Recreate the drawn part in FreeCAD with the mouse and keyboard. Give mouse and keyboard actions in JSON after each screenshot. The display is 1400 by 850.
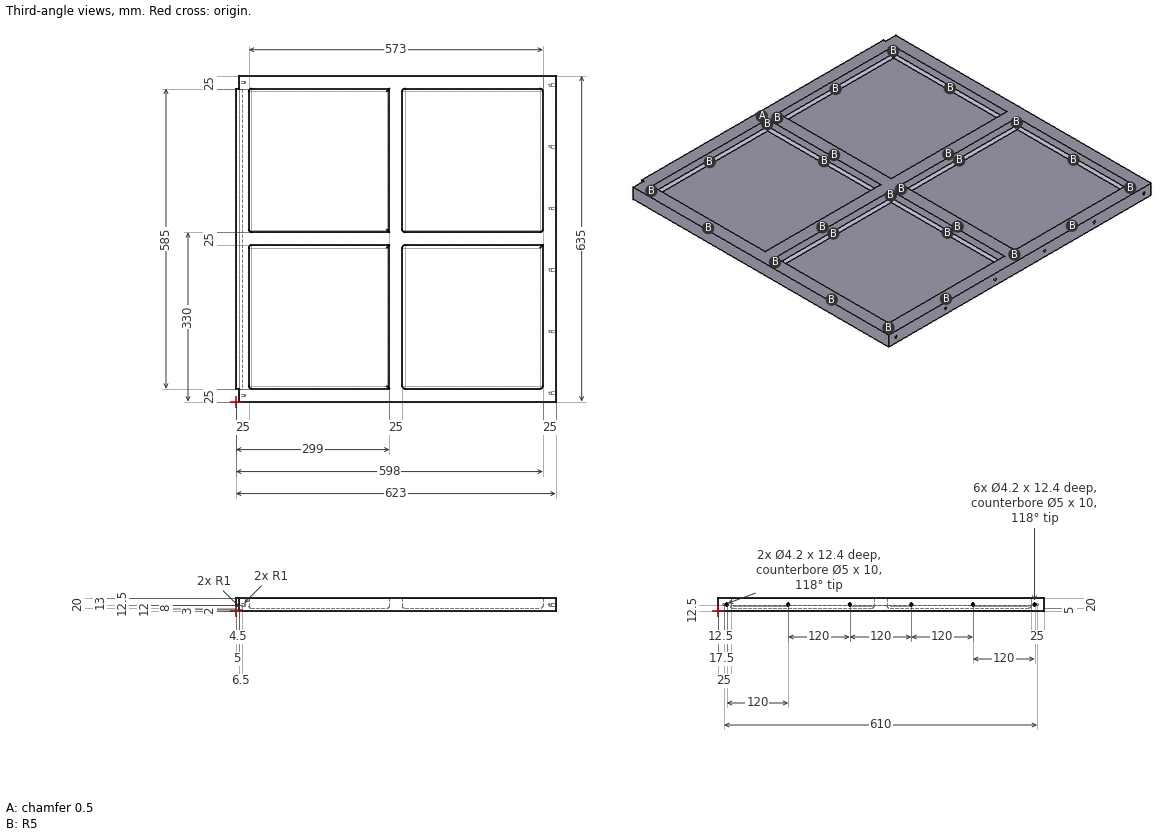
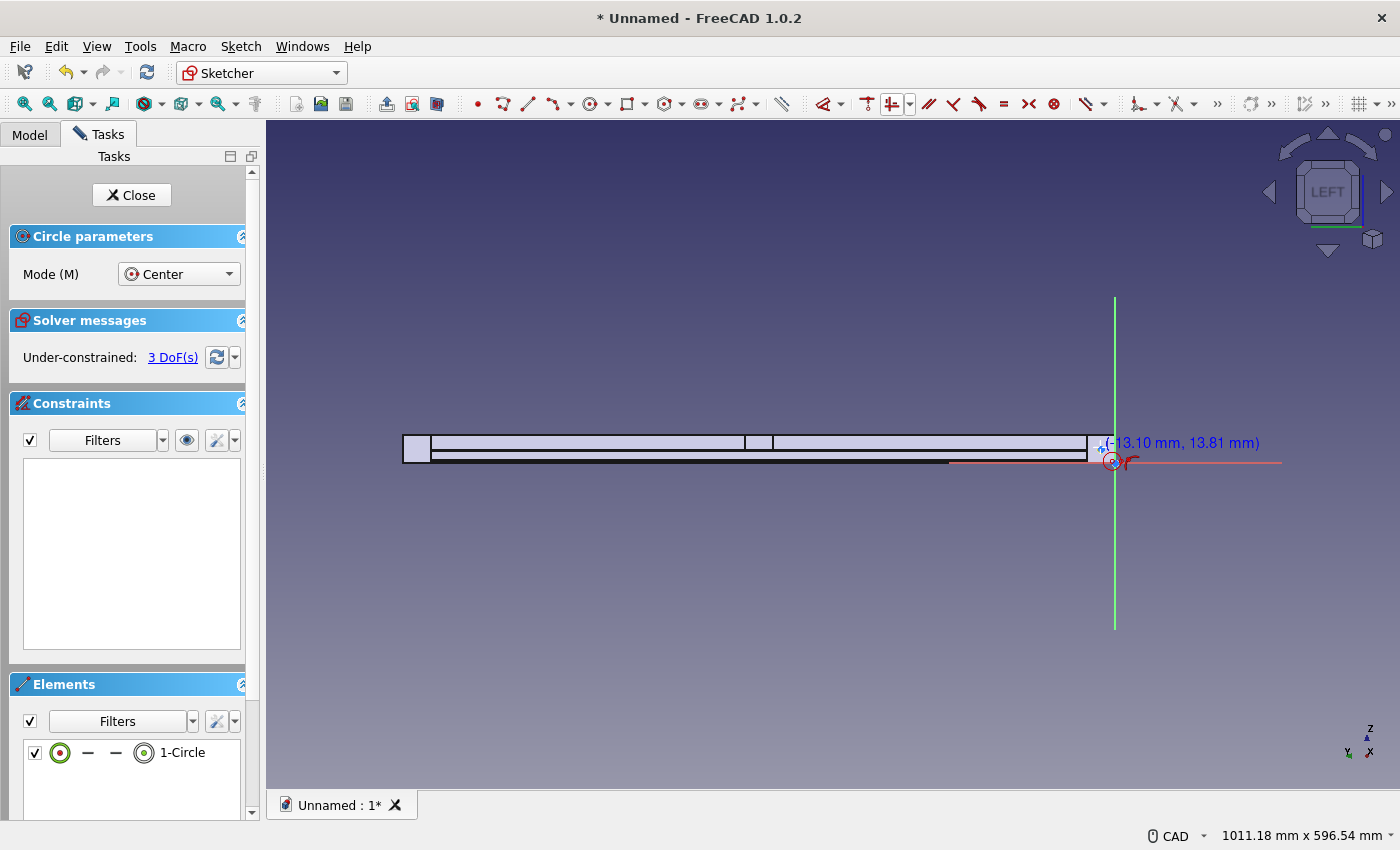
{"action": "scroll", "coordinate": [417, 449], "scroll_direction": "up", "scroll_amount": 12}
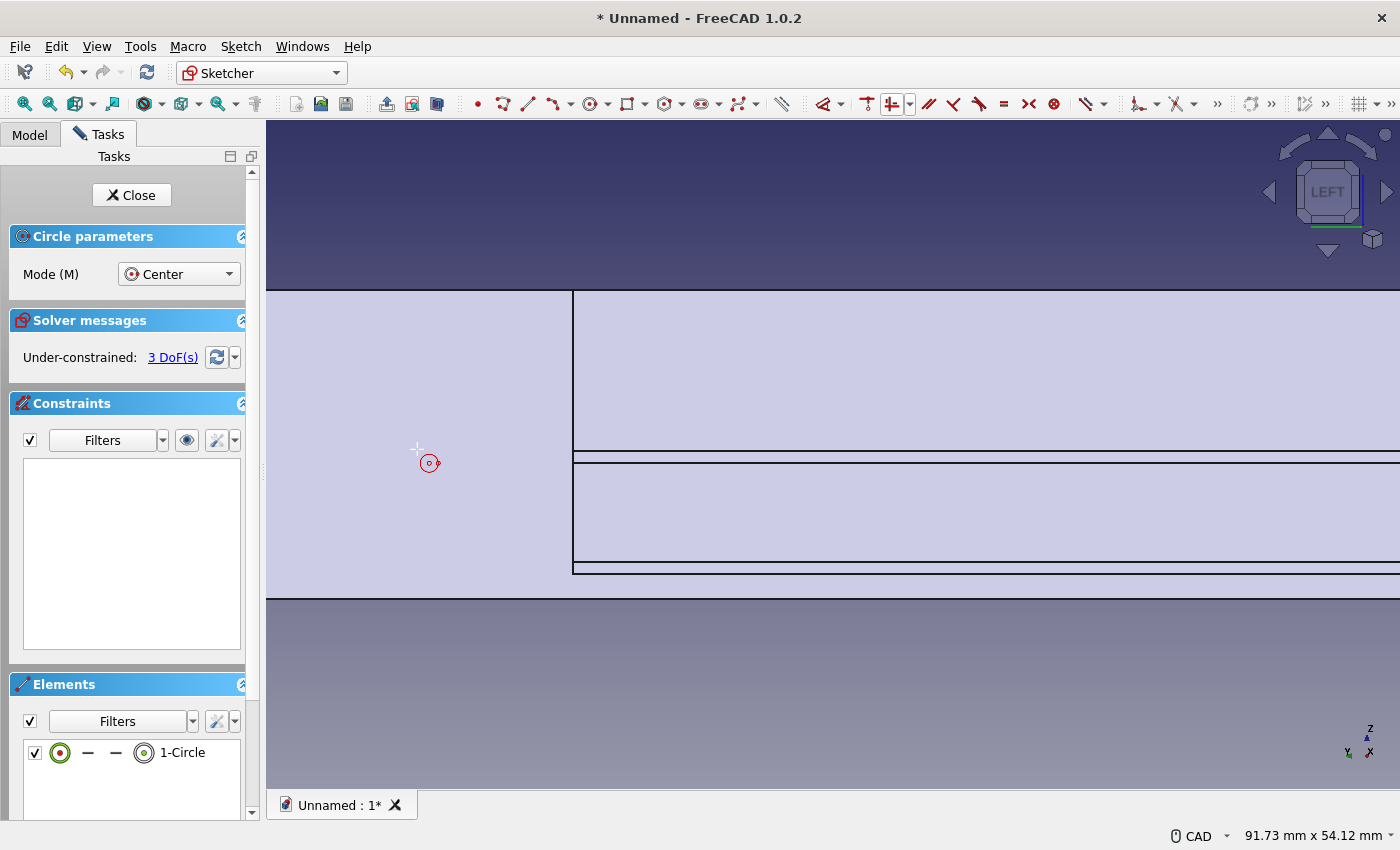
{"action": "scroll", "coordinate": [416, 449], "scroll_direction": "down", "scroll_amount": 12}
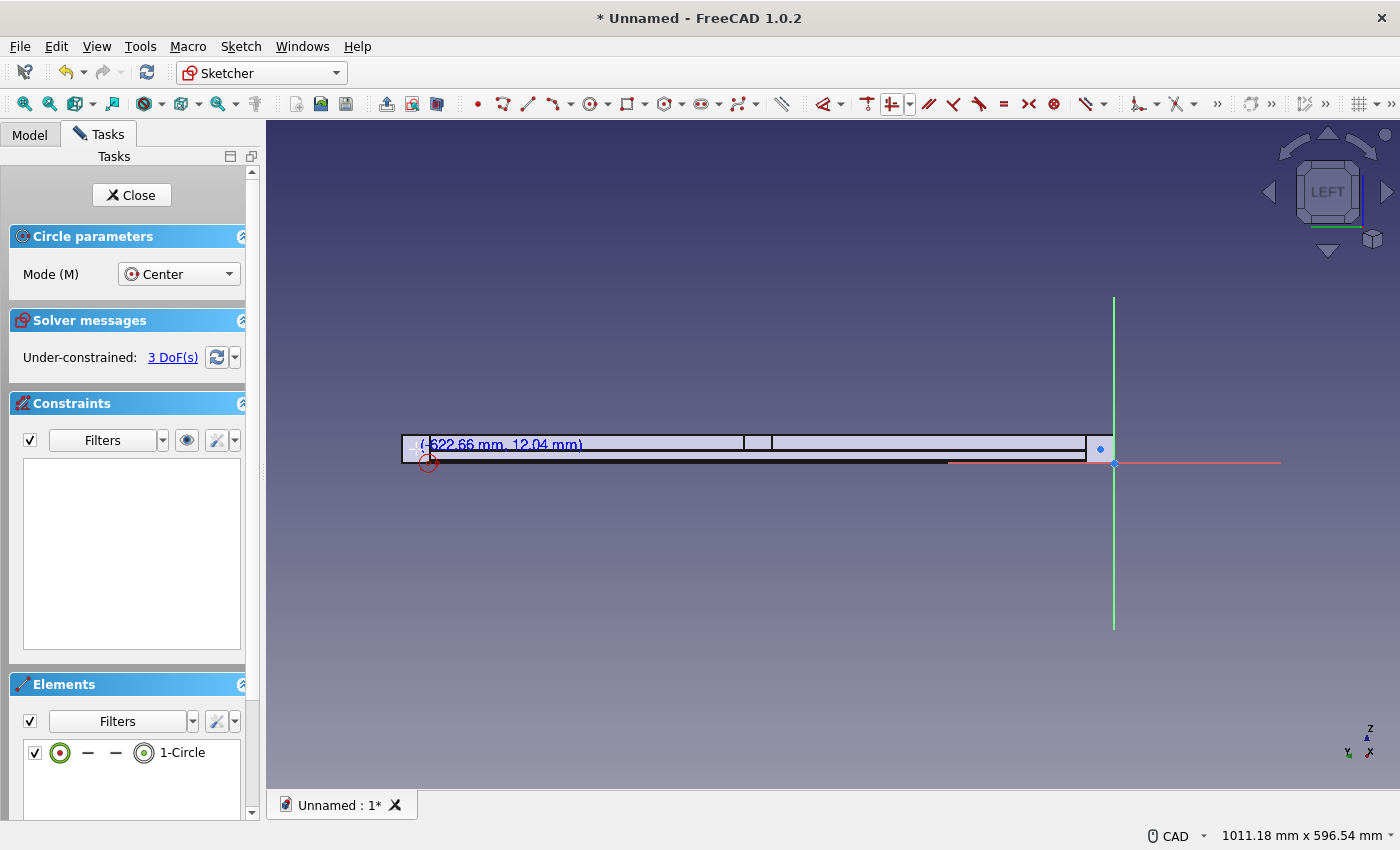
{"action": "left_click", "coordinate": [416, 449]}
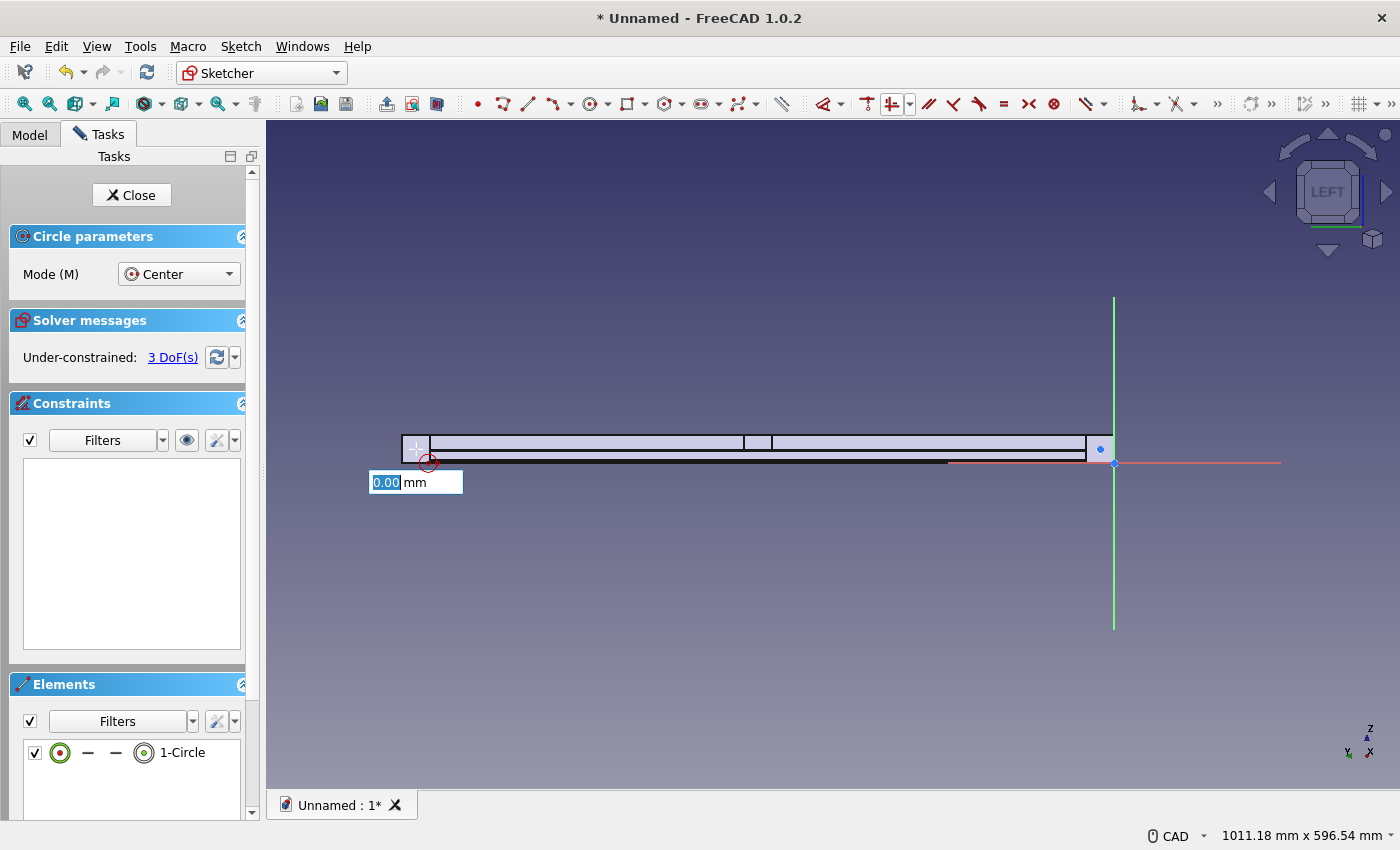
{"action": "scroll", "coordinate": [418, 447], "scroll_direction": "up", "scroll_amount": 10}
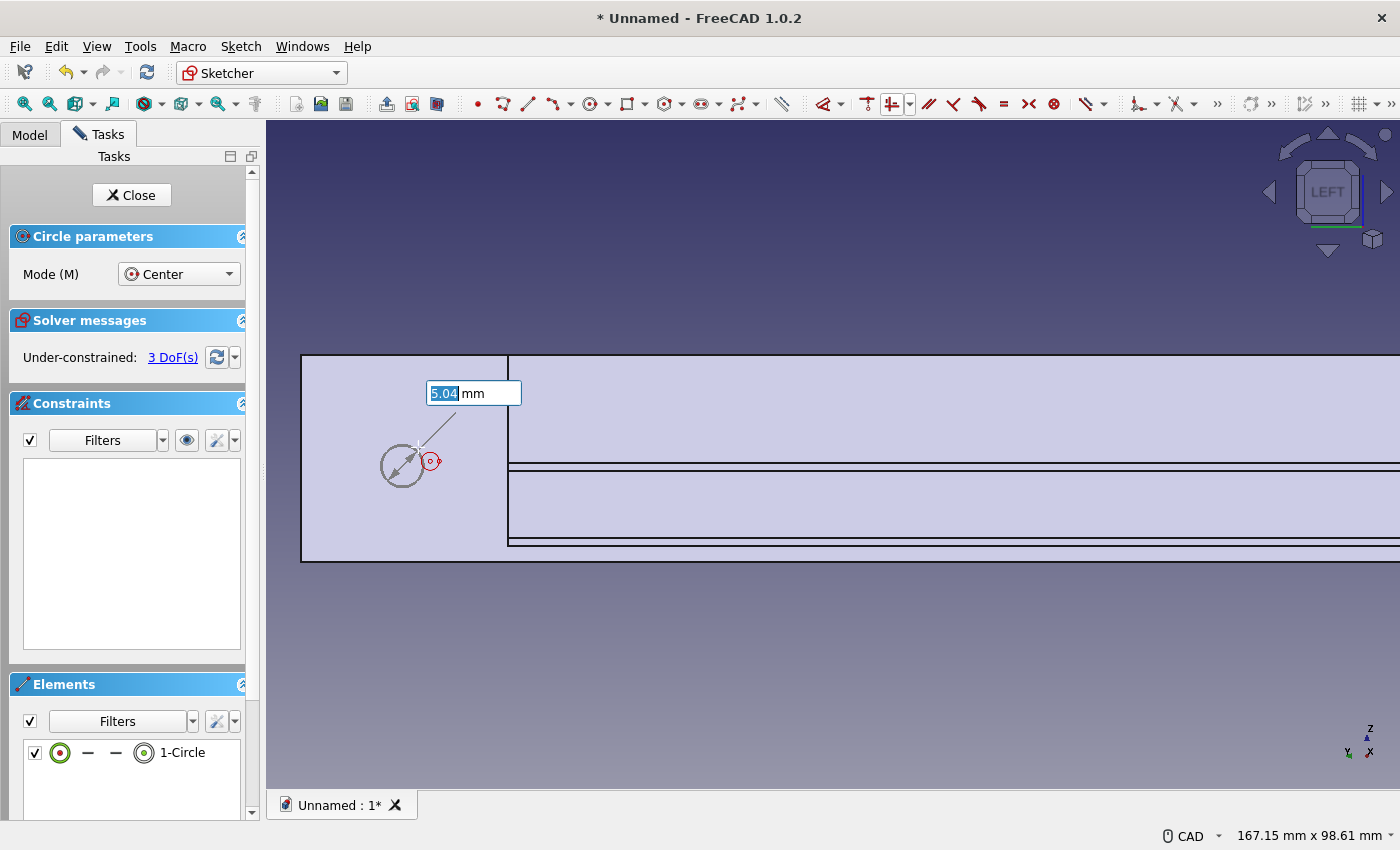
{"action": "left_click", "coordinate": [417, 447]}
{"action": "key", "text": "Escape"}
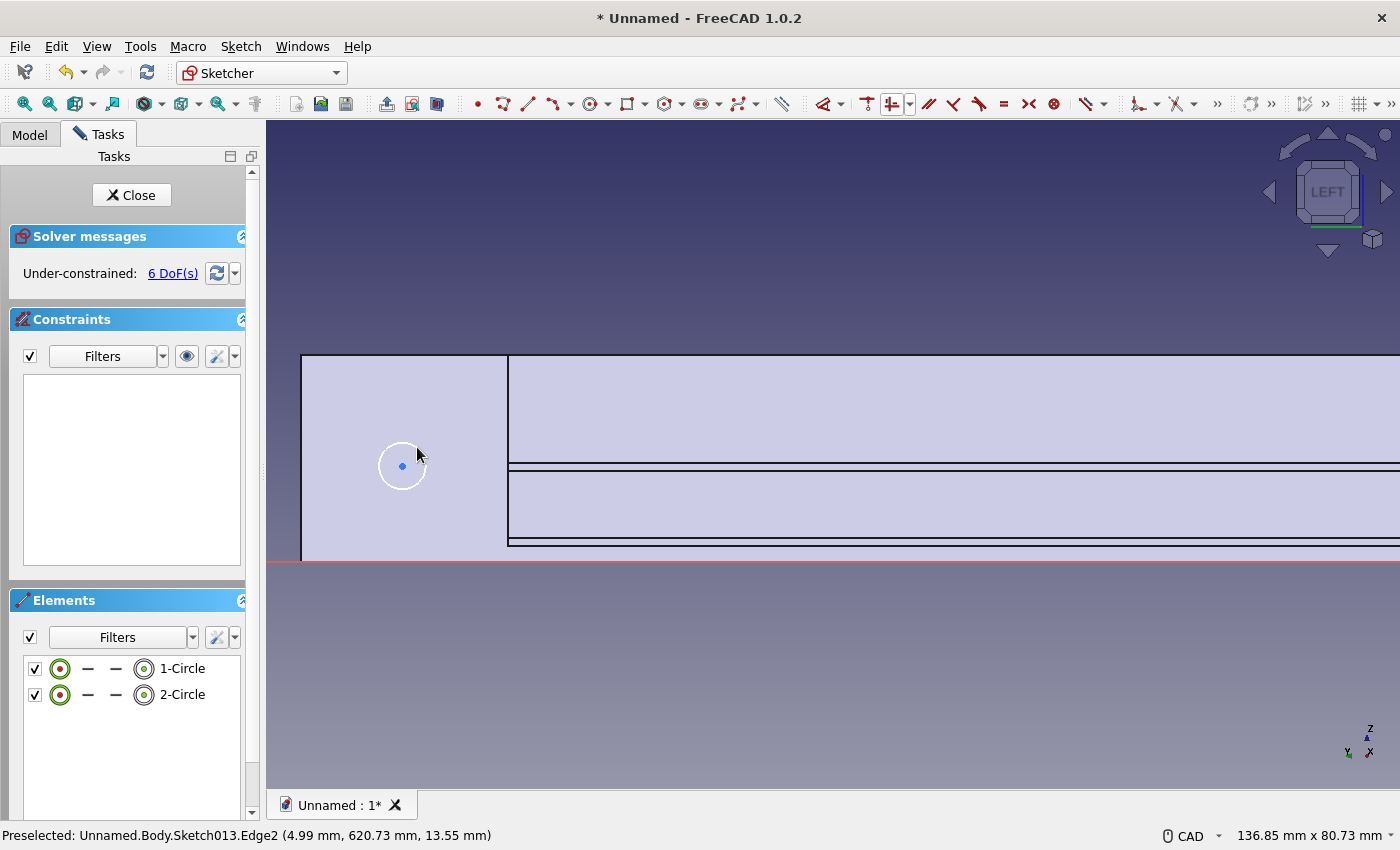
{"action": "scroll", "coordinate": [419, 447], "scroll_direction": "down", "scroll_amount": 10}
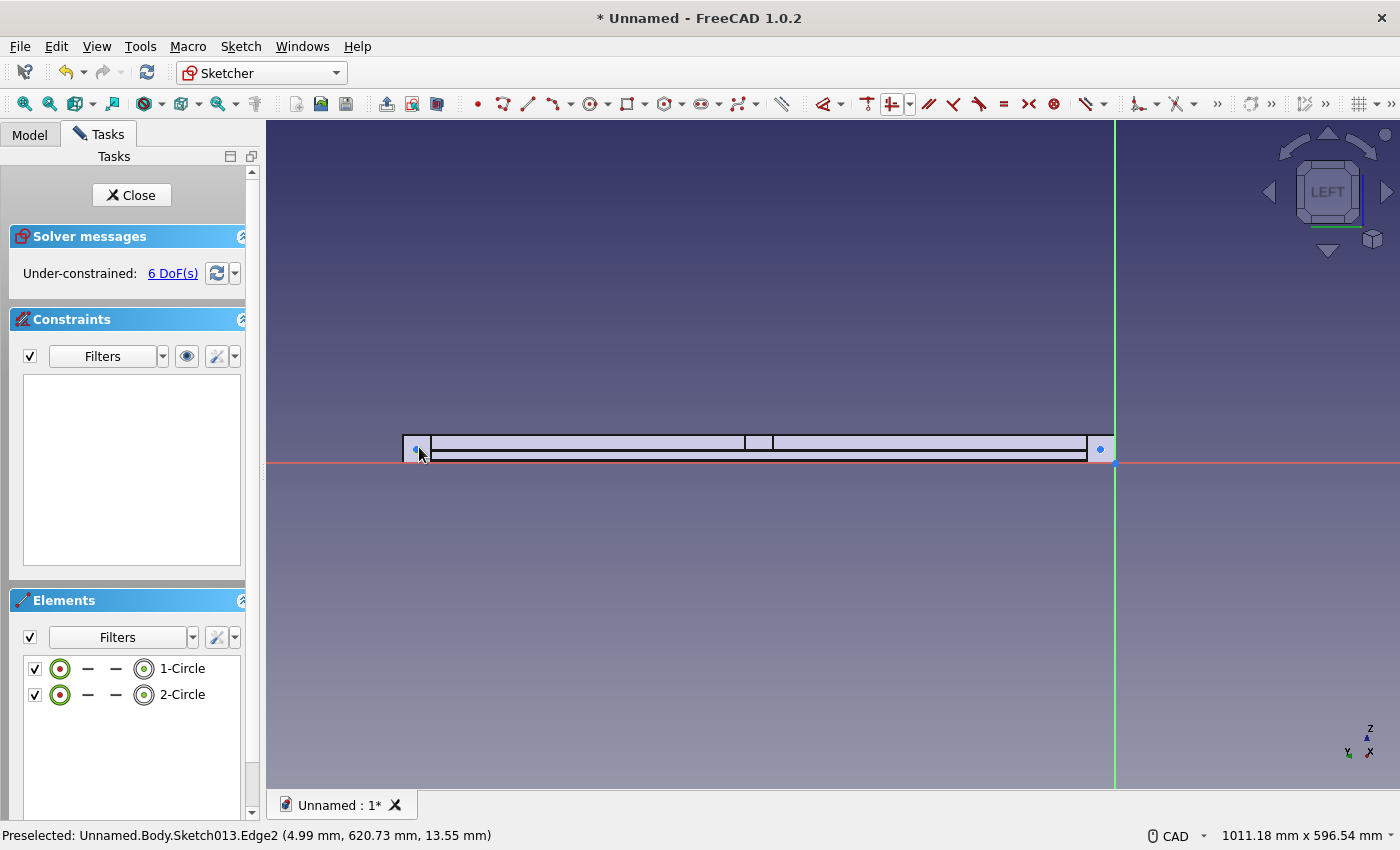
{"action": "scroll", "coordinate": [1103, 448], "scroll_direction": "up", "scroll_amount": 9}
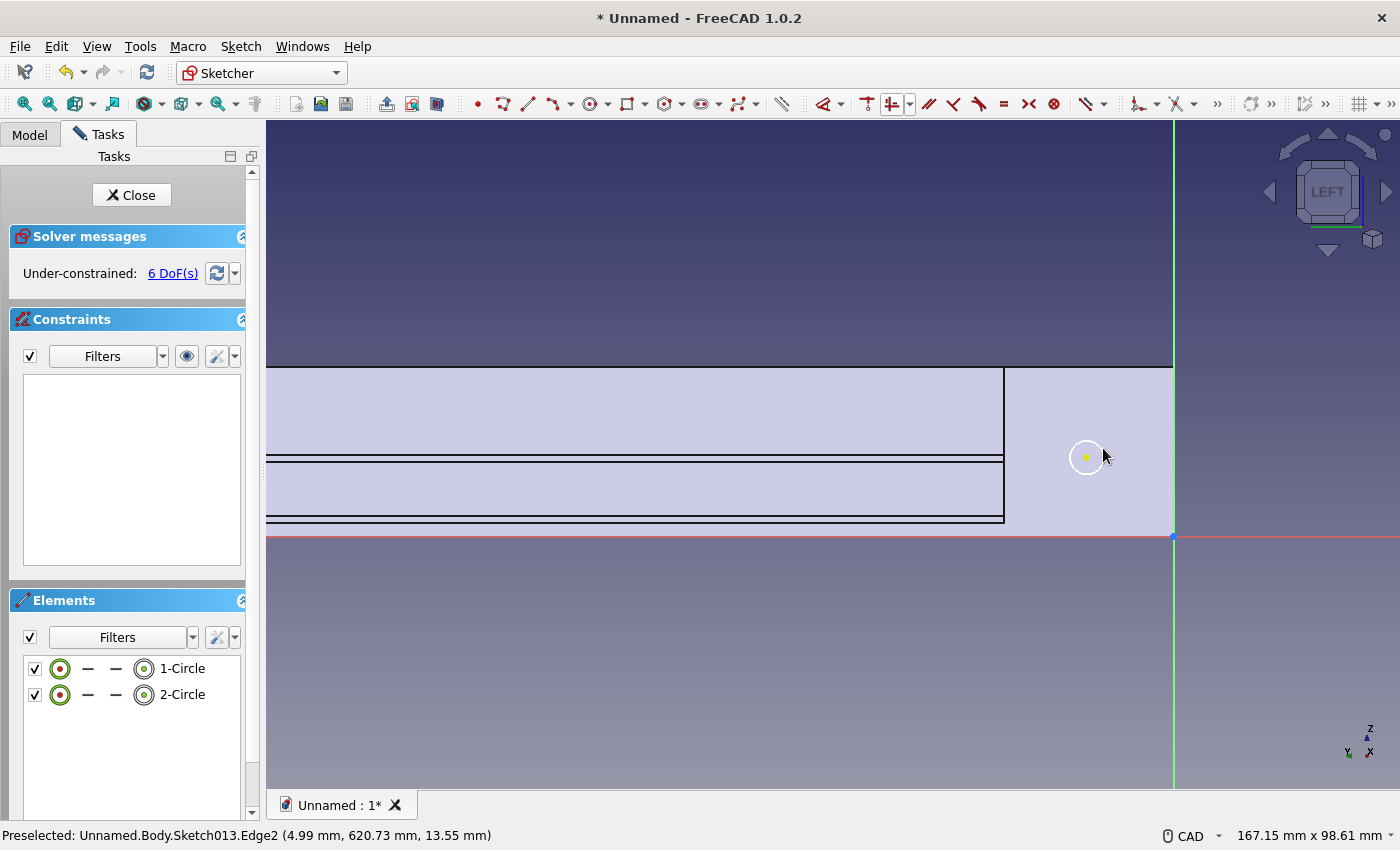
{"action": "left_click", "coordinate": [1099, 446]}